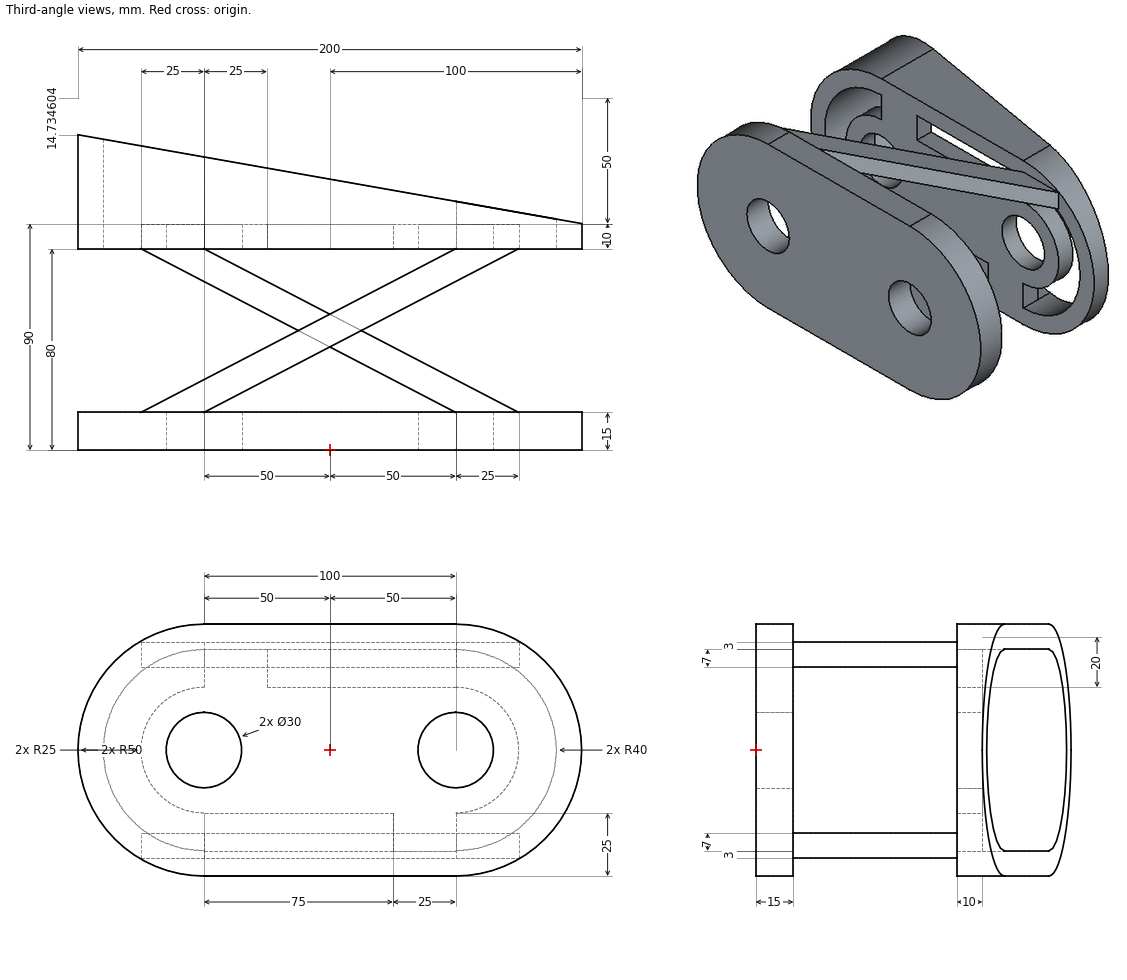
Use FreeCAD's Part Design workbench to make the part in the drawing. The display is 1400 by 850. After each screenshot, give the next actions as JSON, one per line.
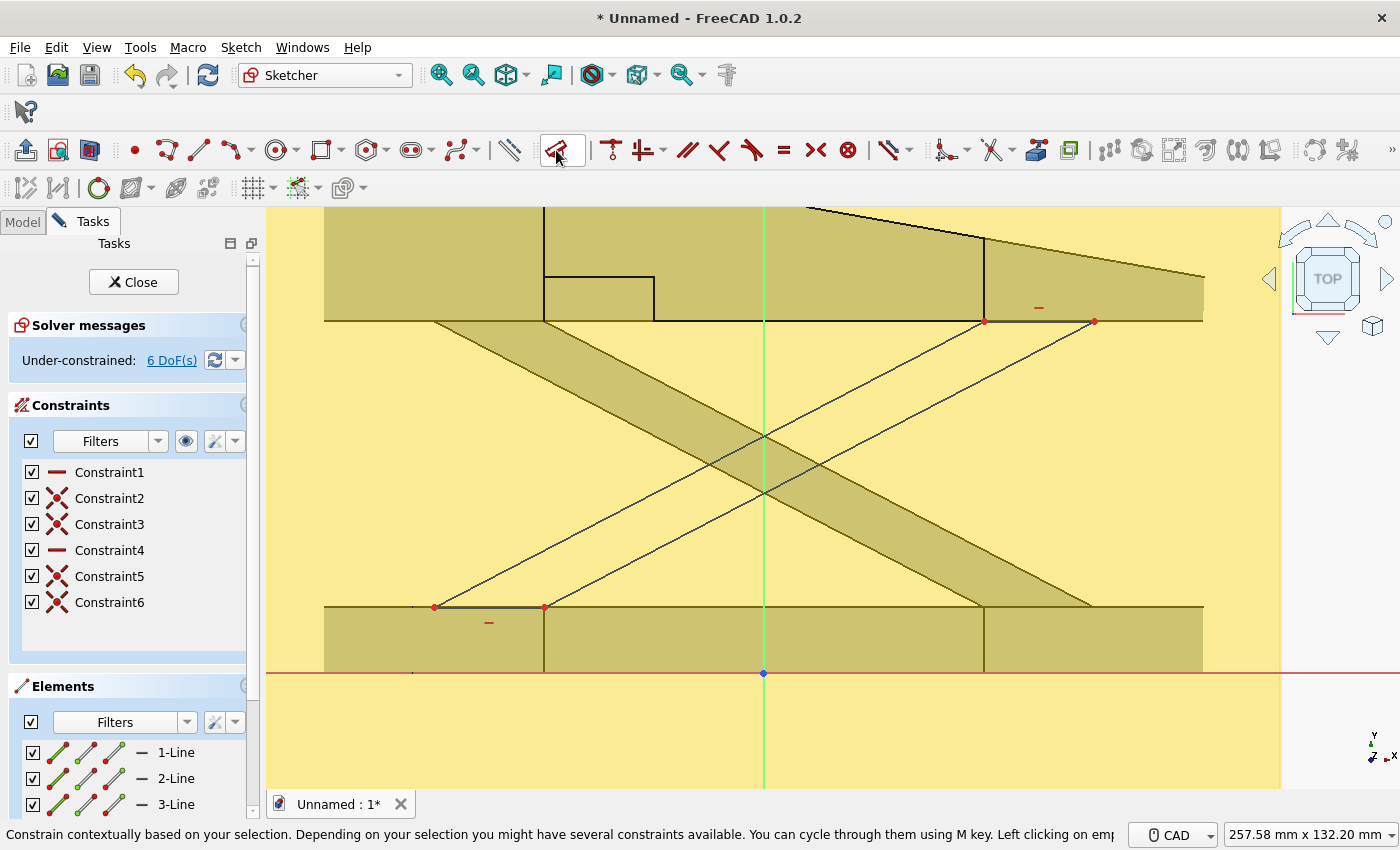
{"action": "left_click", "coordinate": [511, 608]}
{"action": "left_click", "coordinate": [489, 642]}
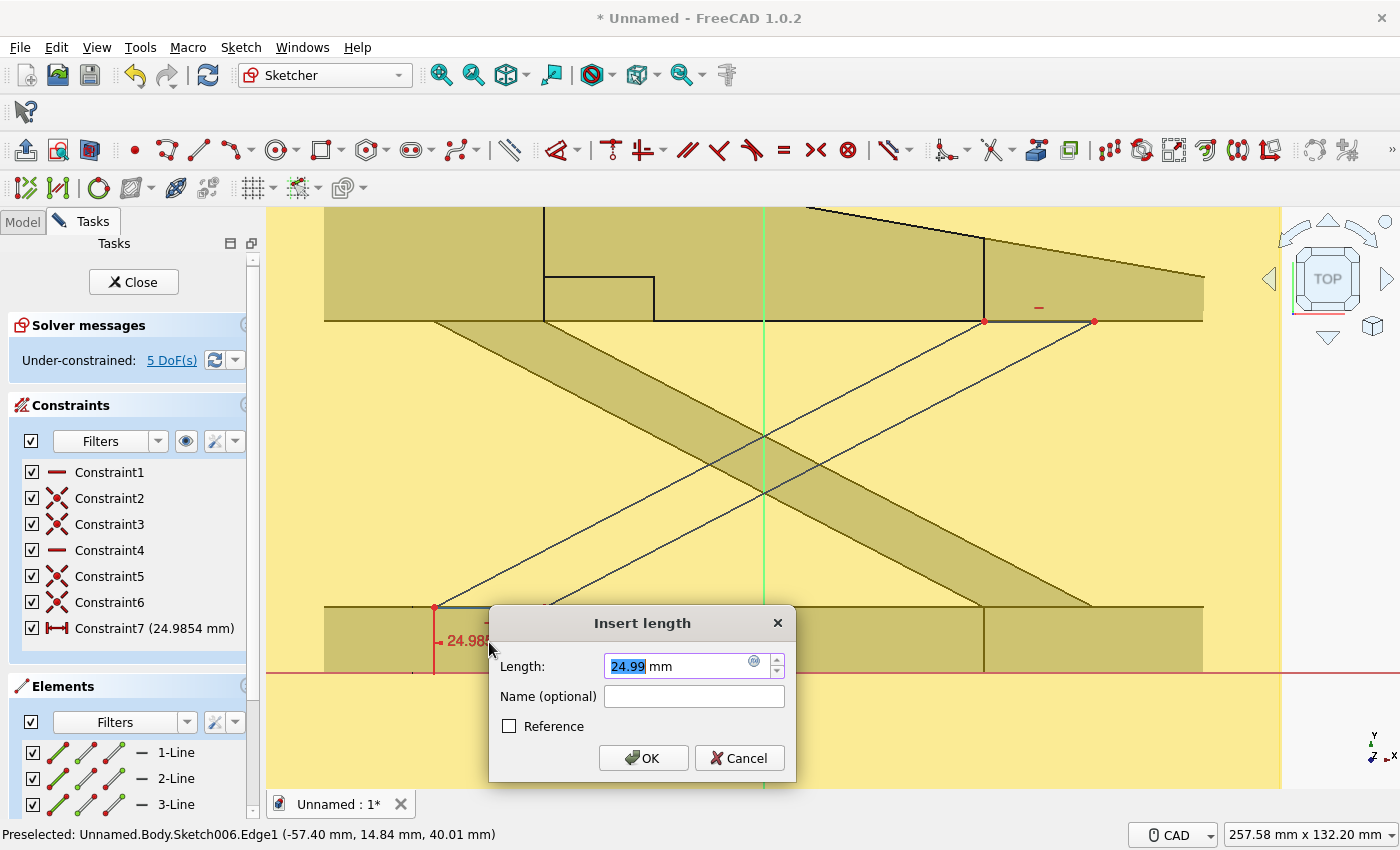
{"action": "type", "text": "25"}
{"action": "key", "text": "Return"}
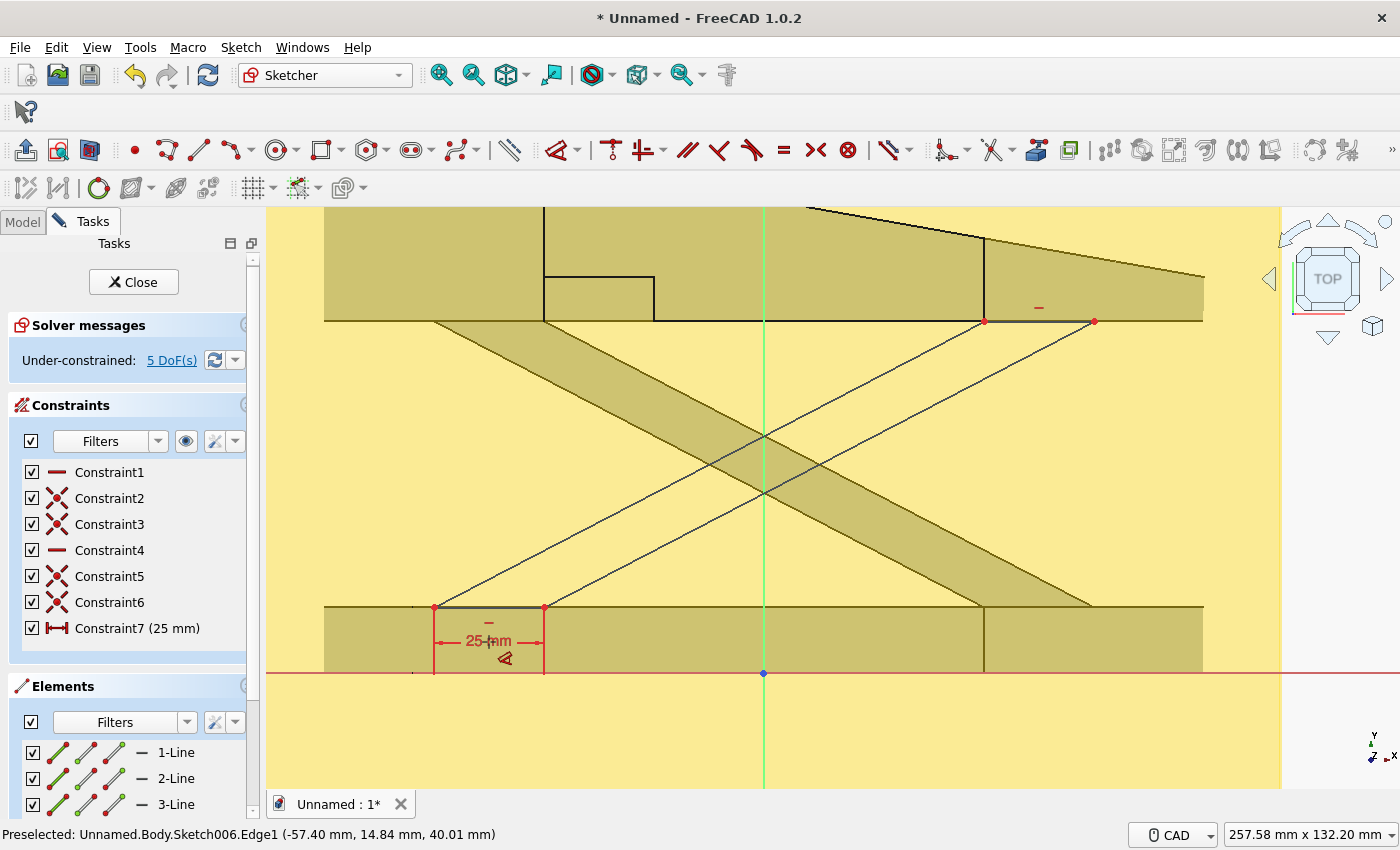
{"action": "left_click", "coordinate": [1017, 322]}
{"action": "left_click", "coordinate": [1039, 288]}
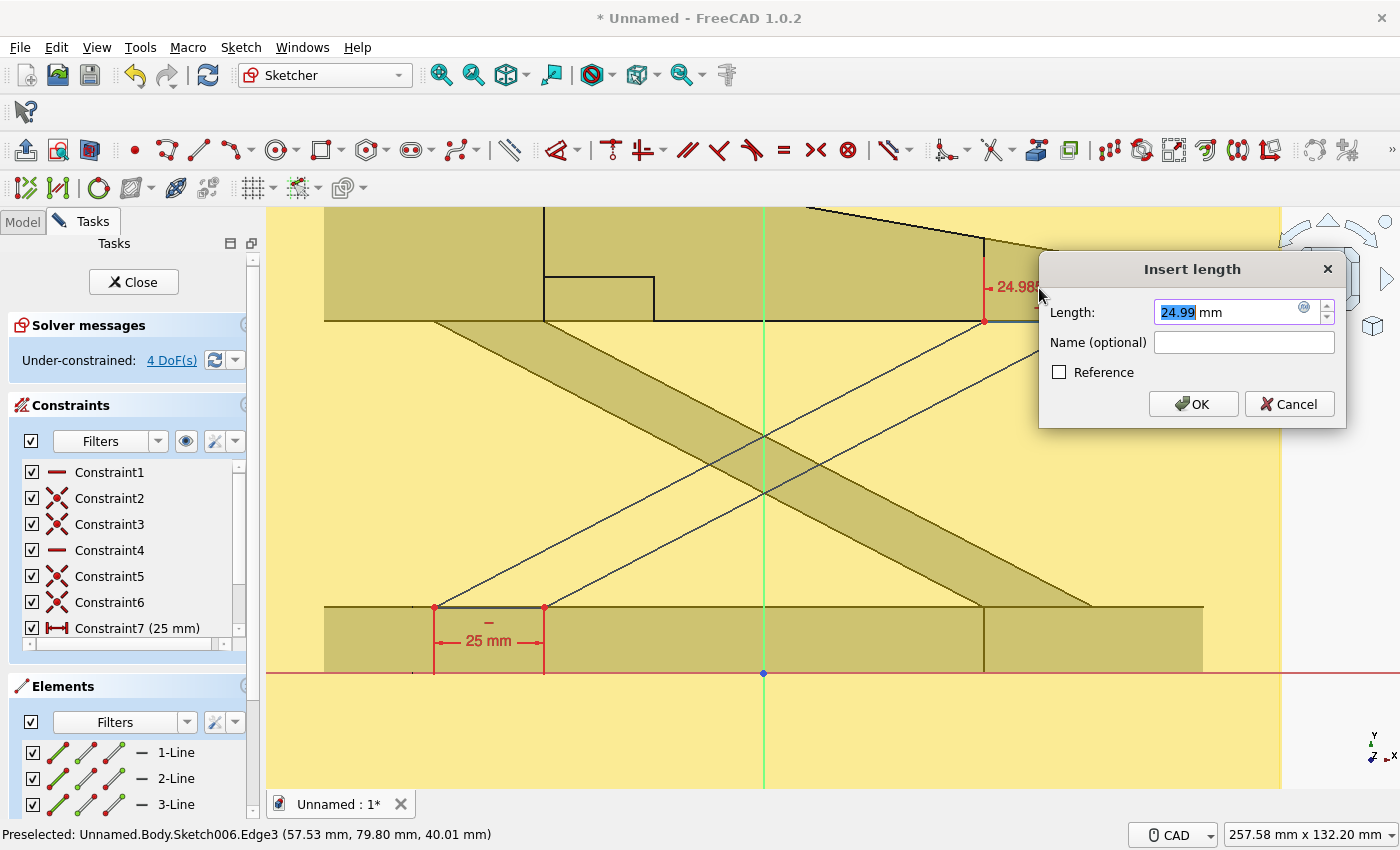
{"action": "type", "text": "25"}
{"action": "key", "text": "Return"}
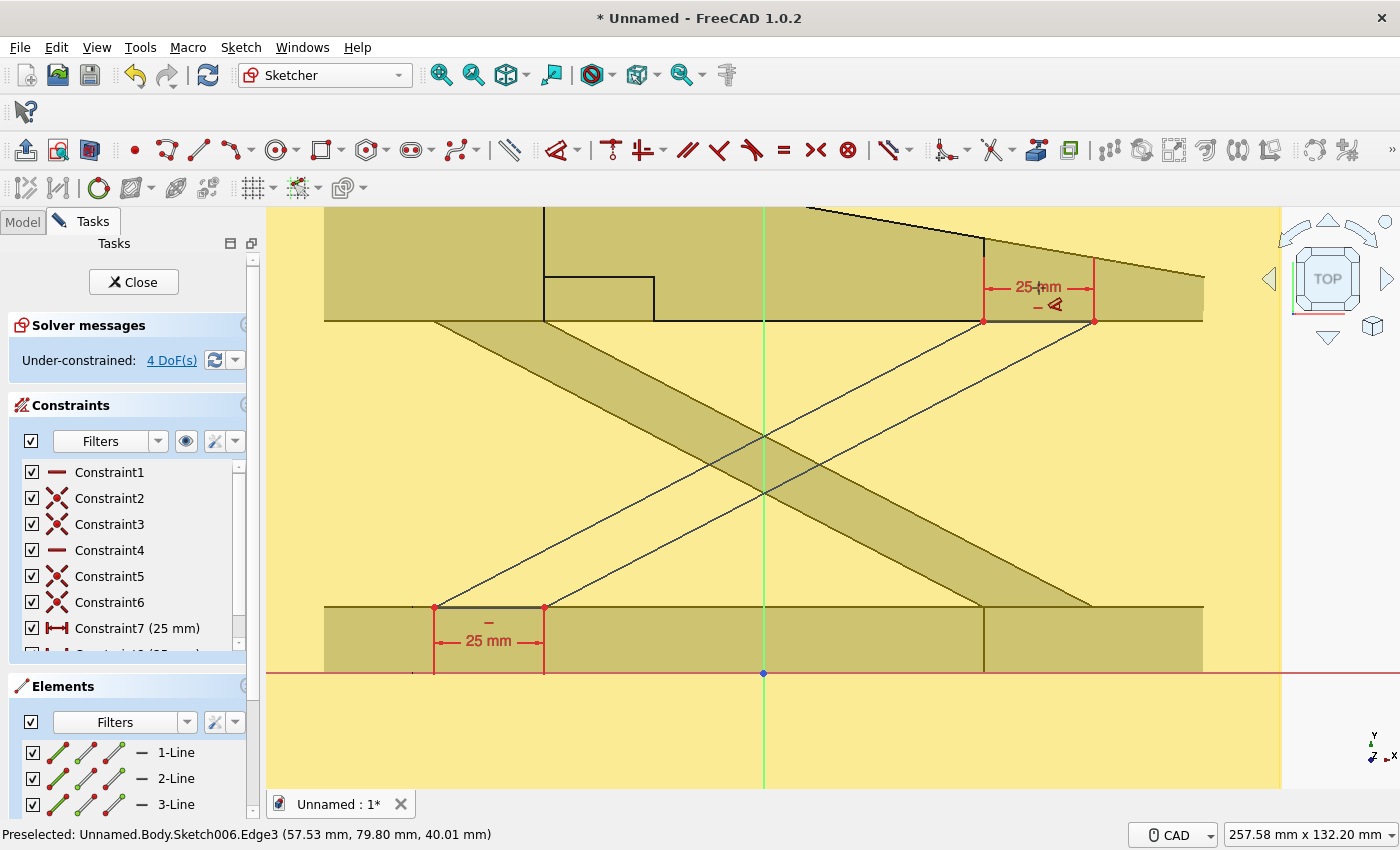
{"action": "left_click", "coordinate": [544, 608]}
{"action": "left_click", "coordinate": [654, 707]}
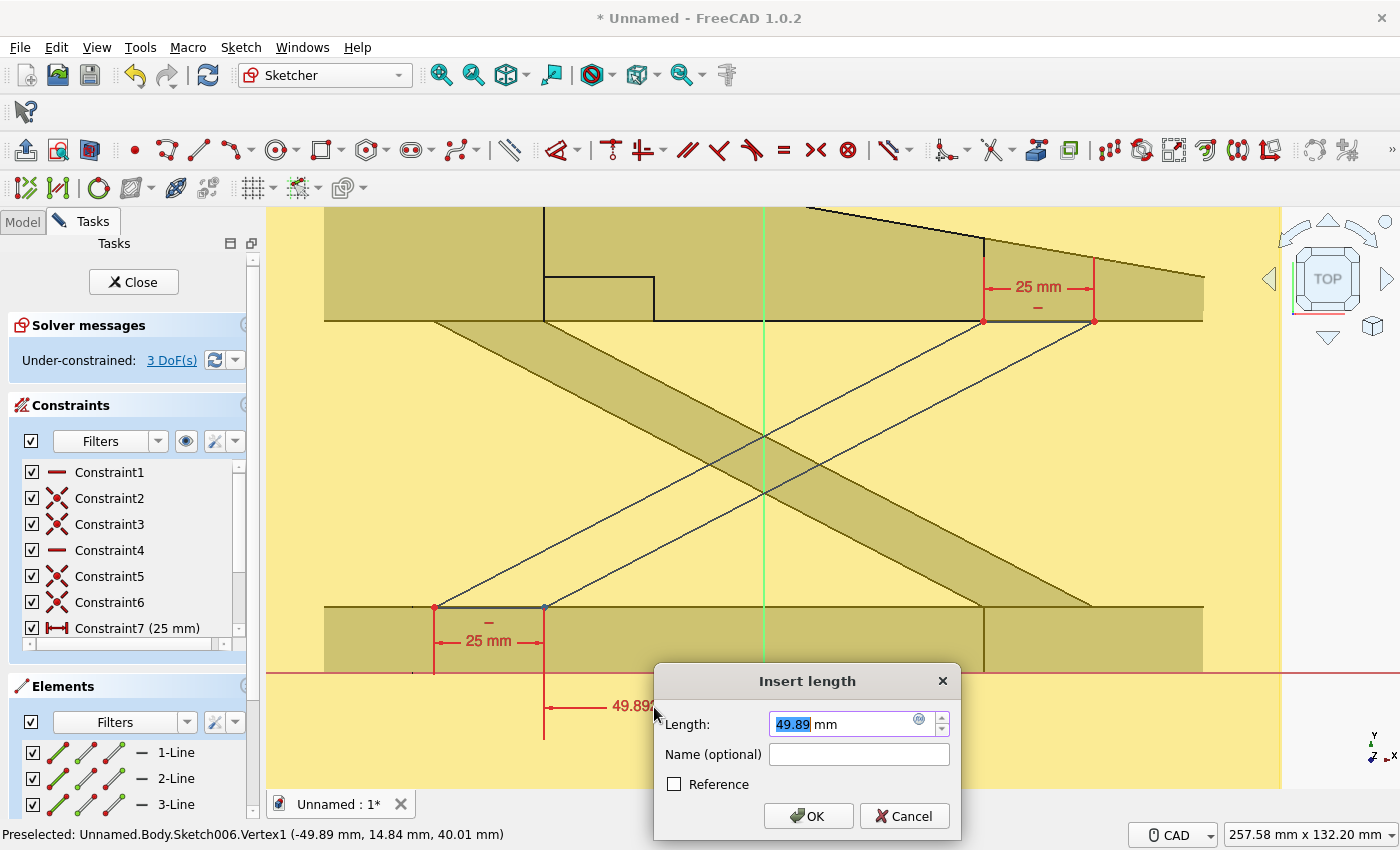
{"action": "type", "text": "50"}
{"action": "key", "text": "Return"}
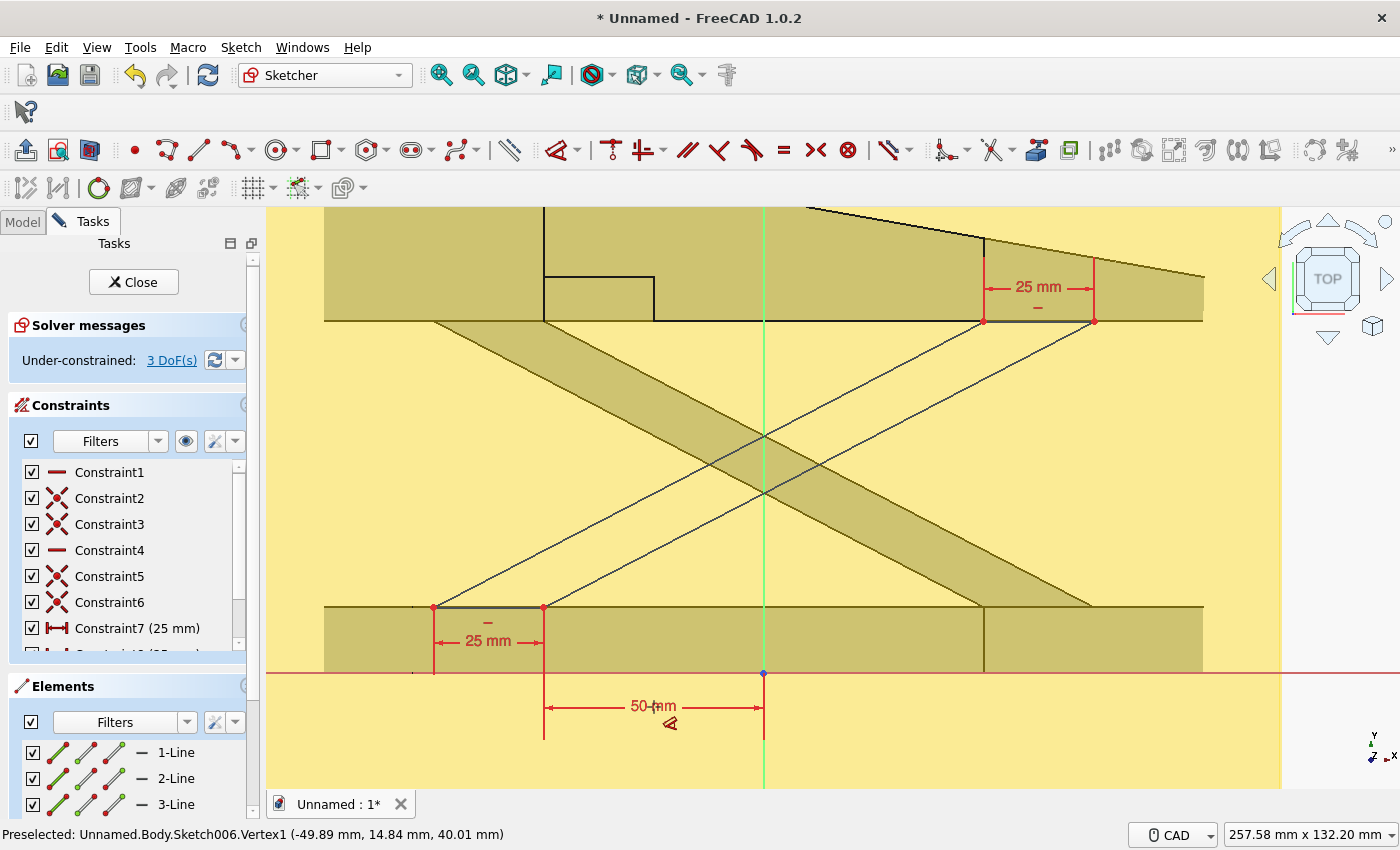
{"action": "left_click", "coordinate": [544, 608]}
{"action": "left_click", "coordinate": [798, 641]}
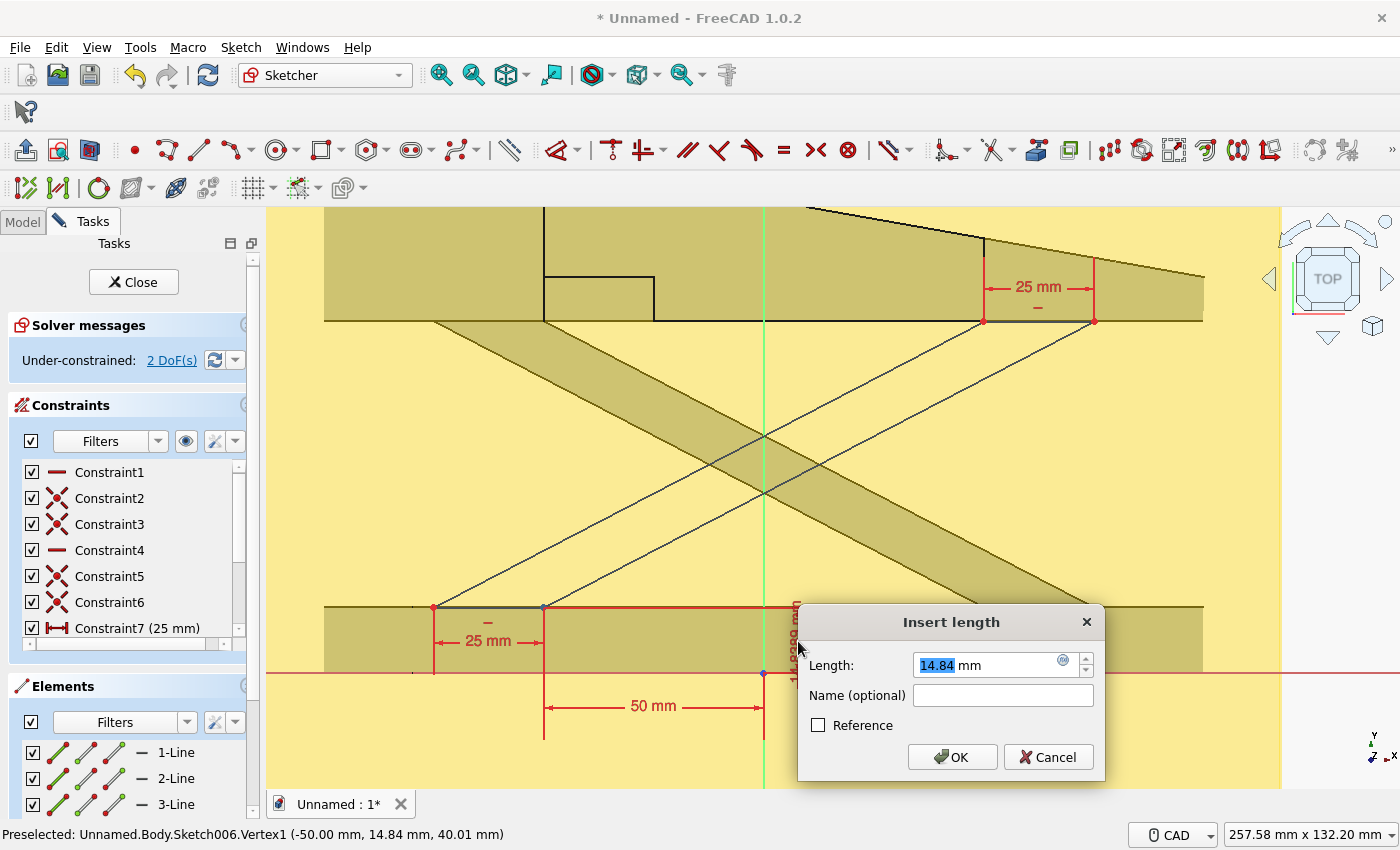
{"action": "type", "text": "15"}
{"action": "key", "text": "Return"}